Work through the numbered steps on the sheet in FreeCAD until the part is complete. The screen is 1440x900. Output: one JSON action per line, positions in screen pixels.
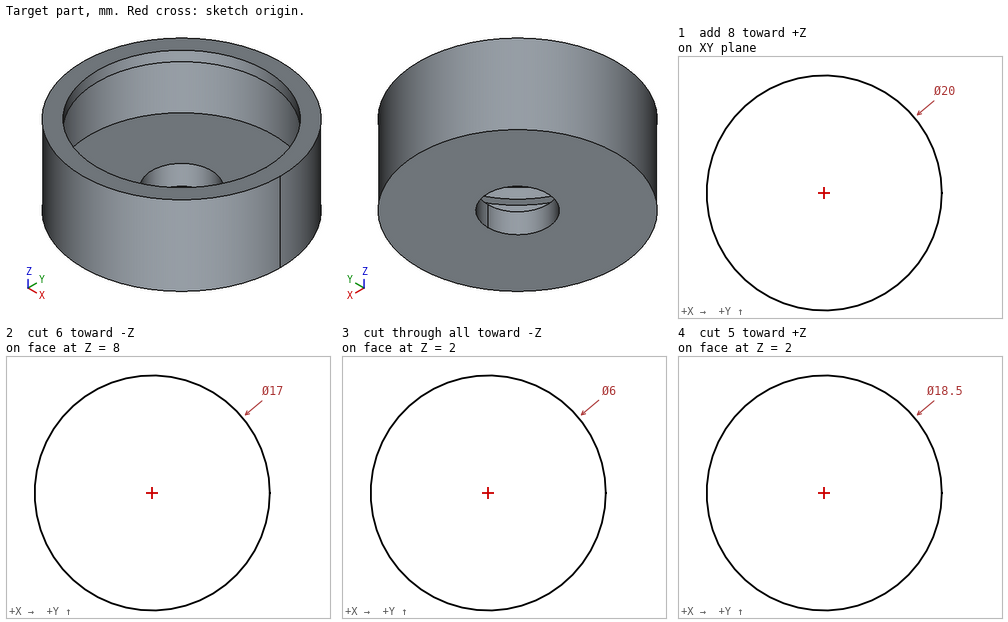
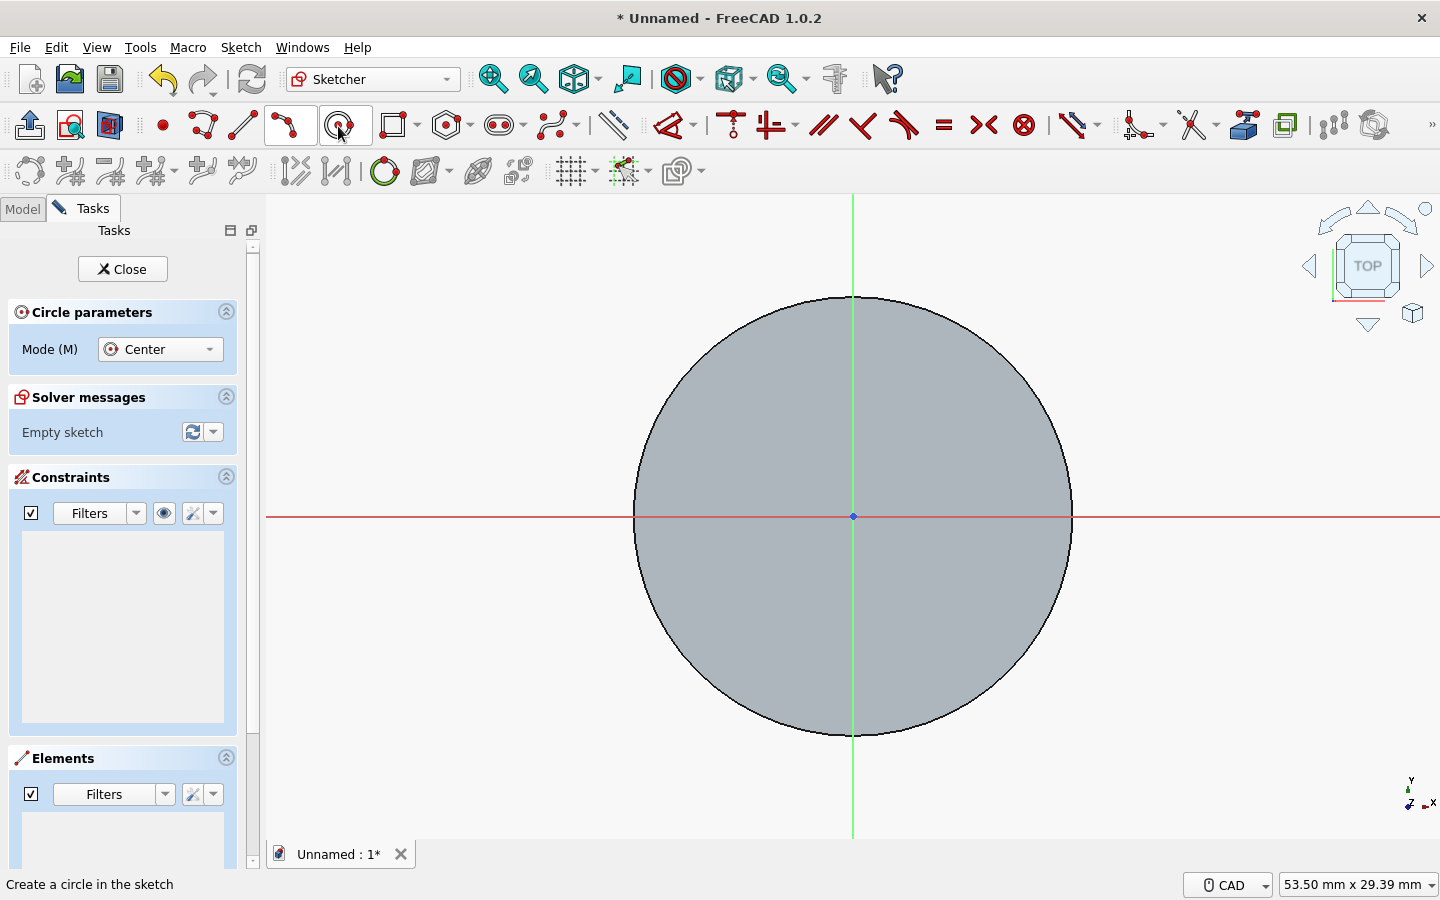
{"action": "left_click", "coordinate": [853, 516]}
{"action": "mouse_move", "coordinate": [985, 385]}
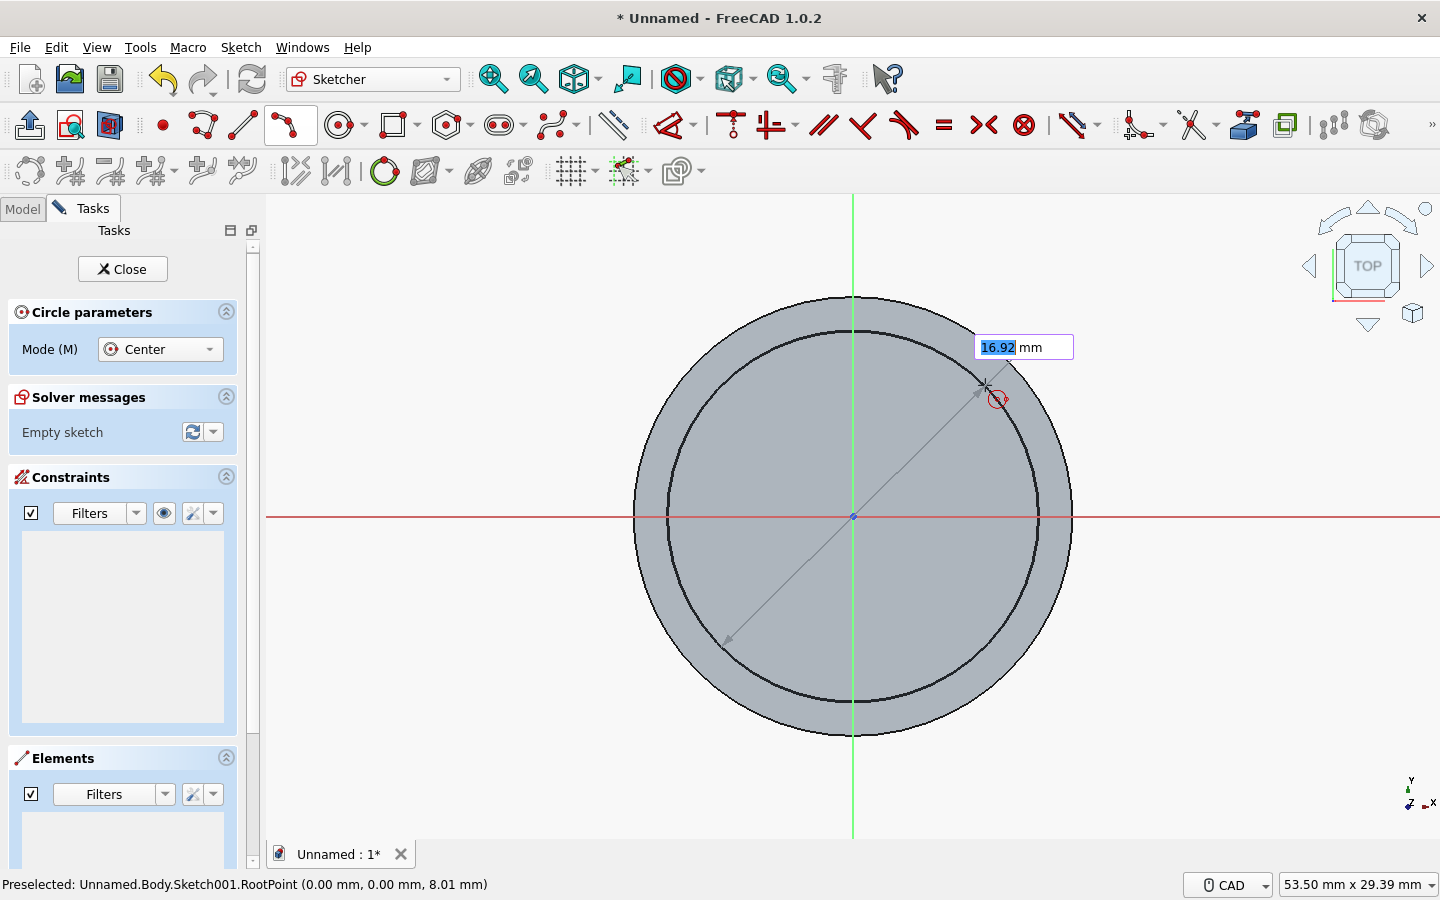
{"action": "type", "text": "17"}
{"action": "key", "text": "Return"}
{"action": "key", "text": "Escape"}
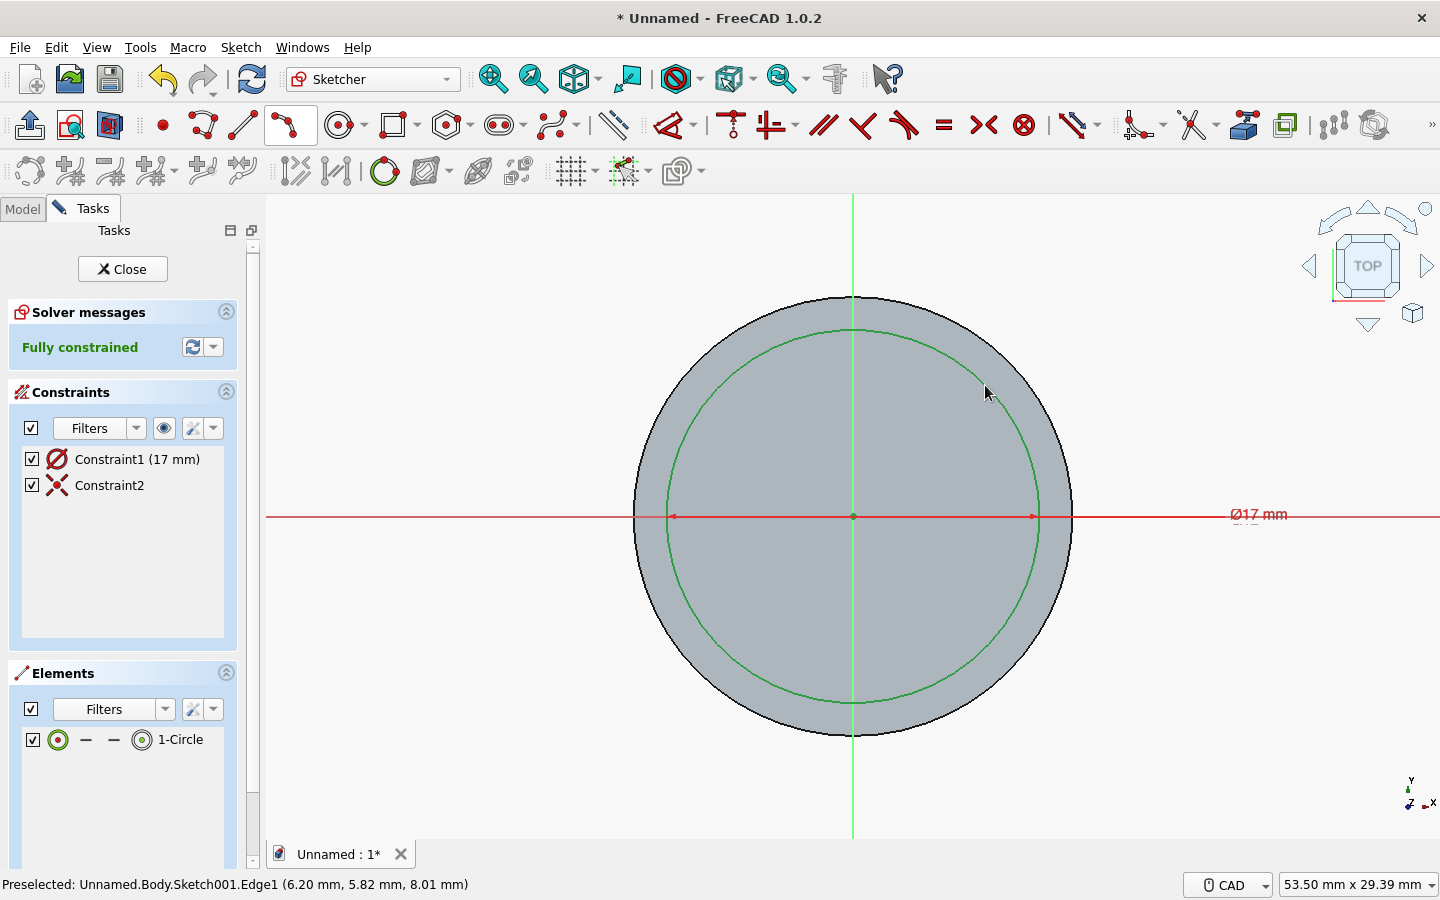
{"action": "left_click", "coordinate": [123, 269]}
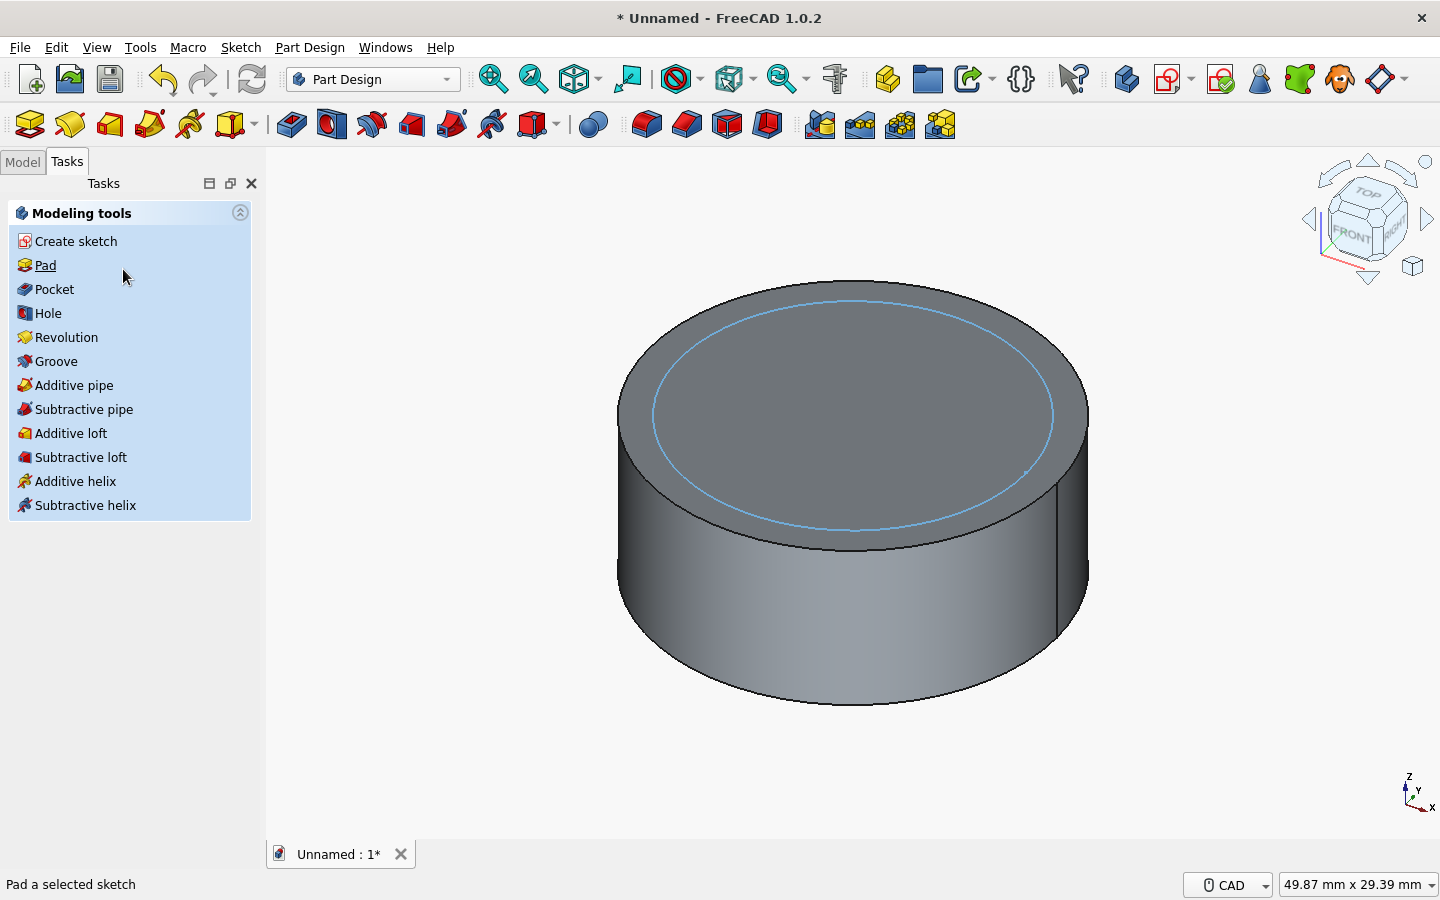
{"action": "left_click", "coordinate": [292, 124]}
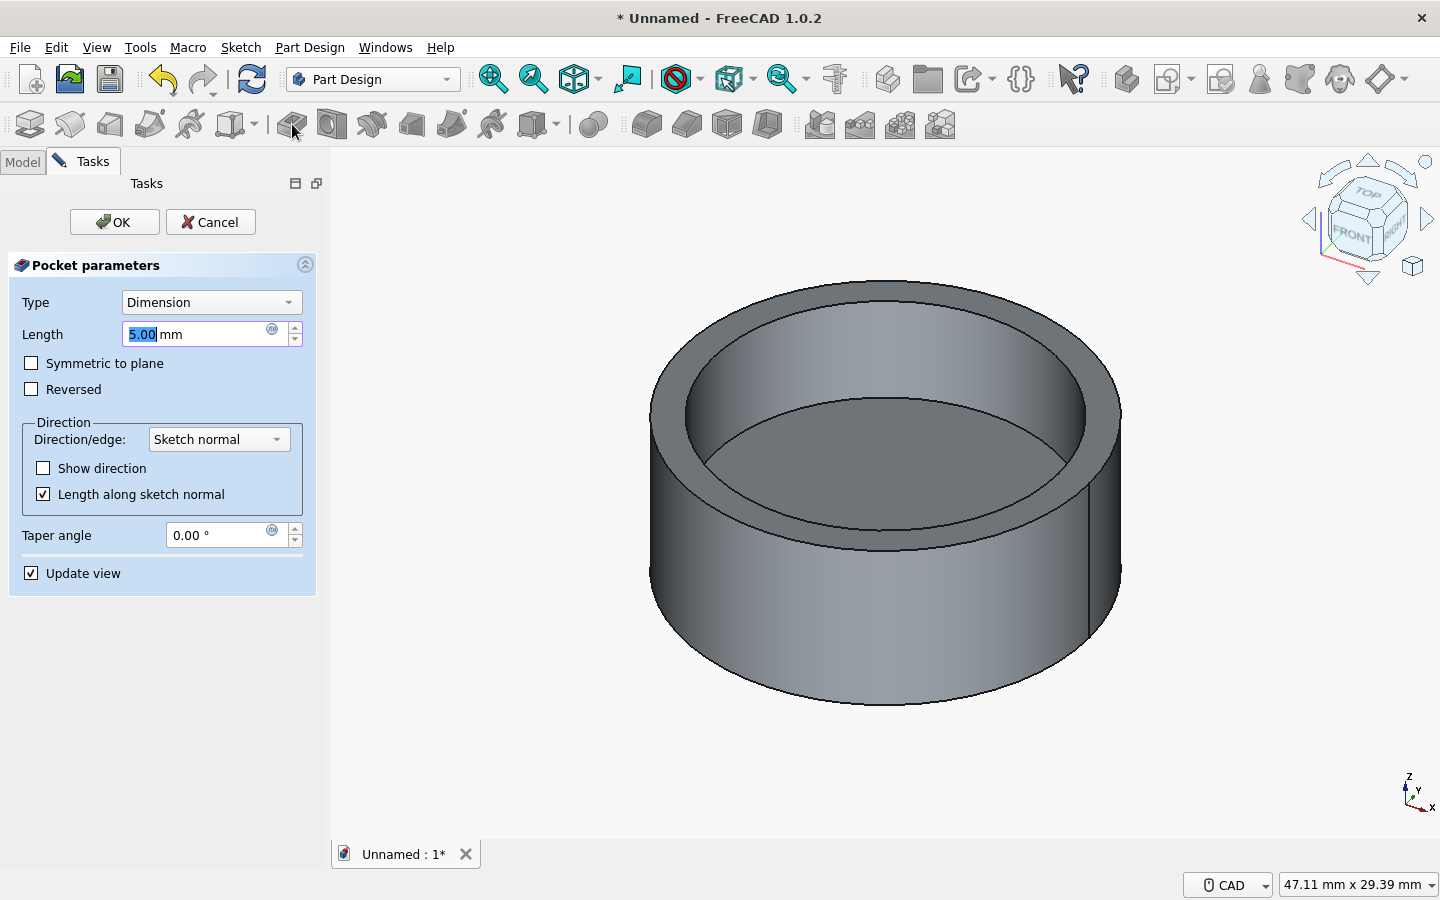
{"action": "type", "text": "6"}
{"action": "key", "text": "Tab"}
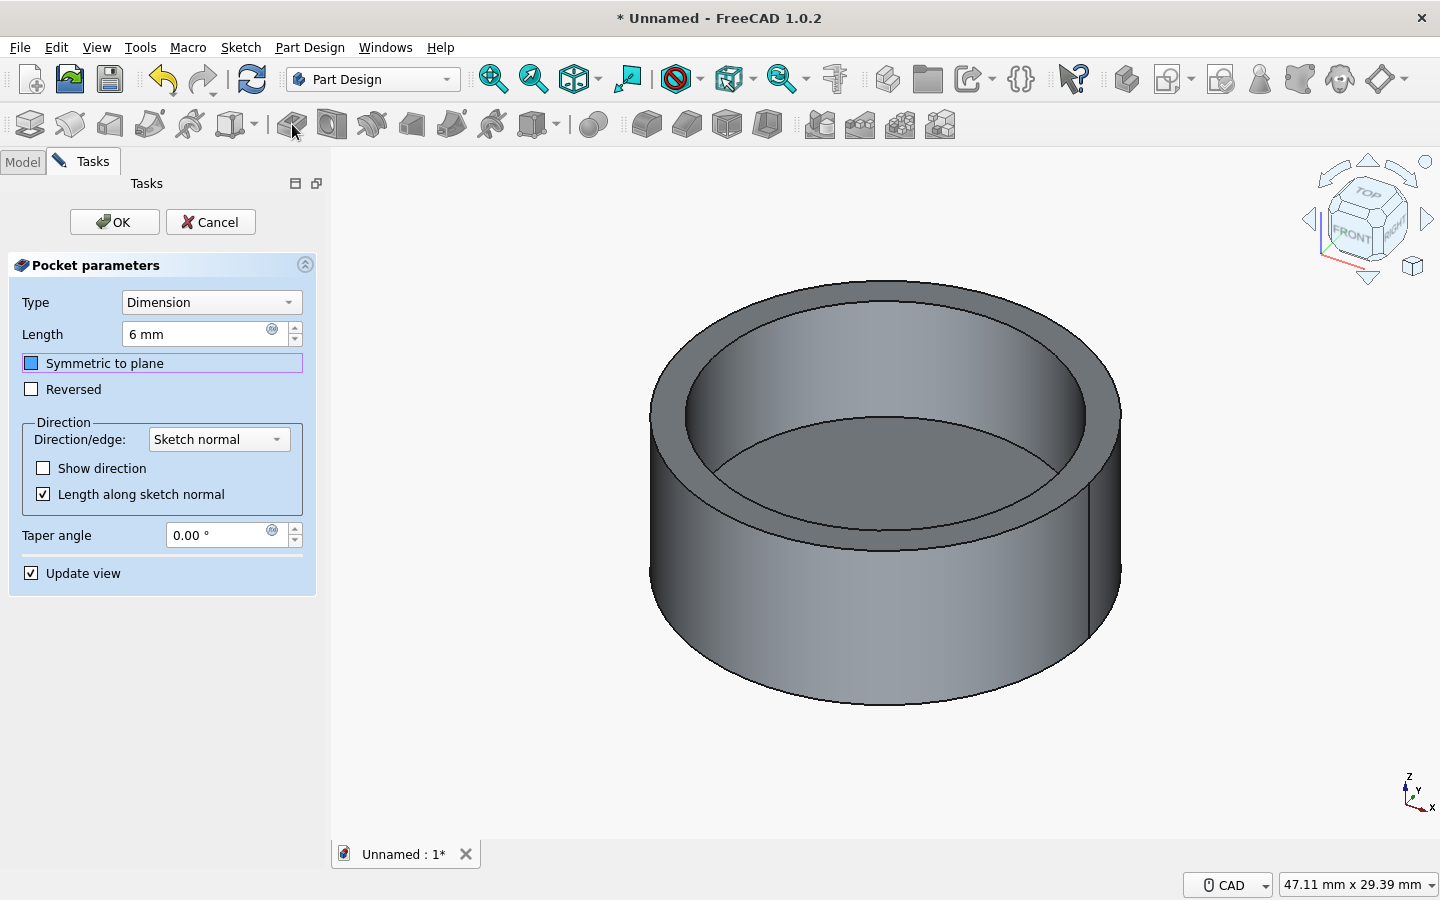
{"action": "left_click", "coordinate": [115, 222]}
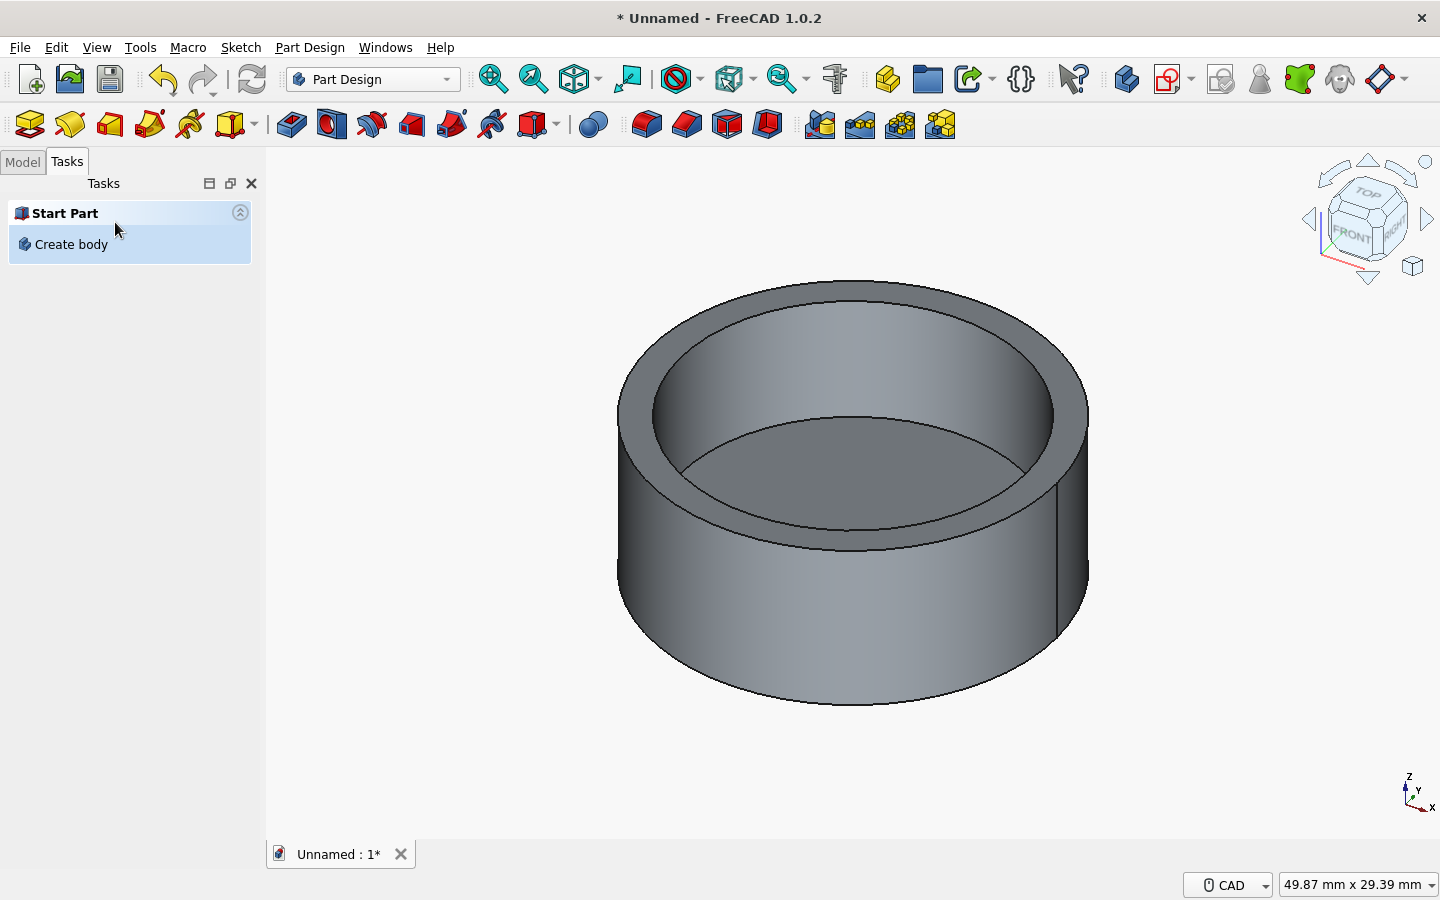
{"action": "left_click", "coordinate": [882, 502]}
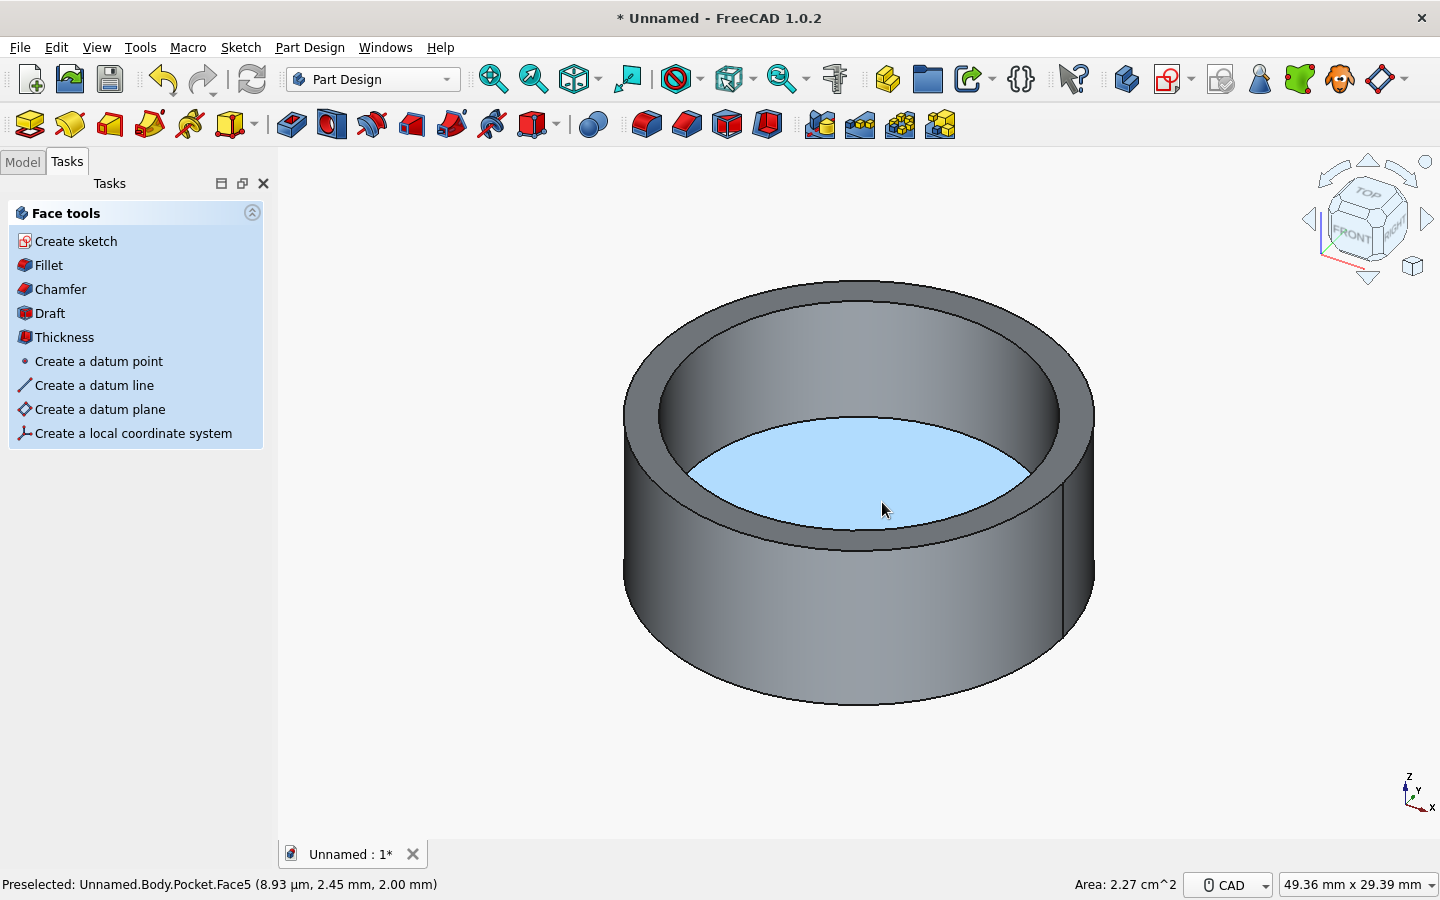
{"action": "left_click", "coordinate": [1168, 80]}